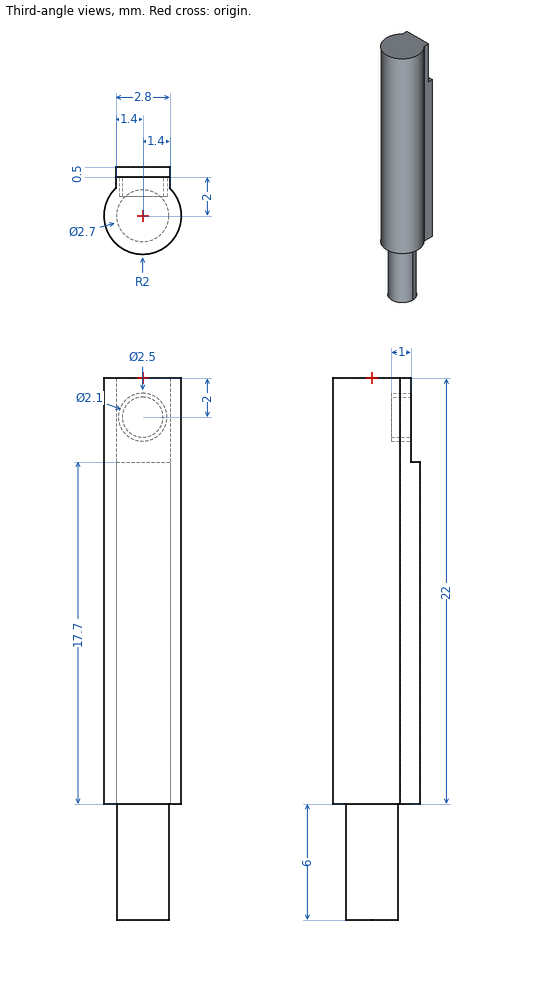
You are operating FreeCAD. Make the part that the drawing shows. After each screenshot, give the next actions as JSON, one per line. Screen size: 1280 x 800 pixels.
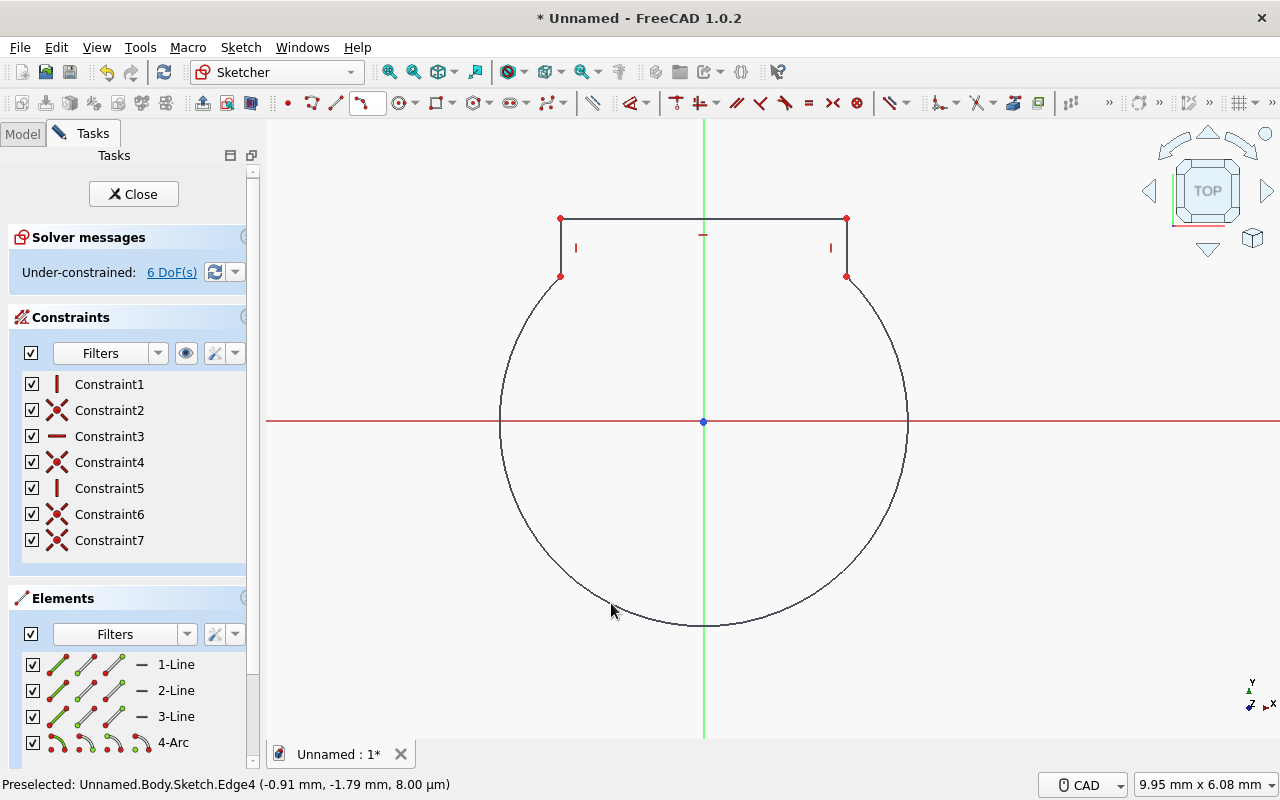
{"action": "left_click_drag", "start_coordinate": [694, 411], "coordinate": [714, 432]}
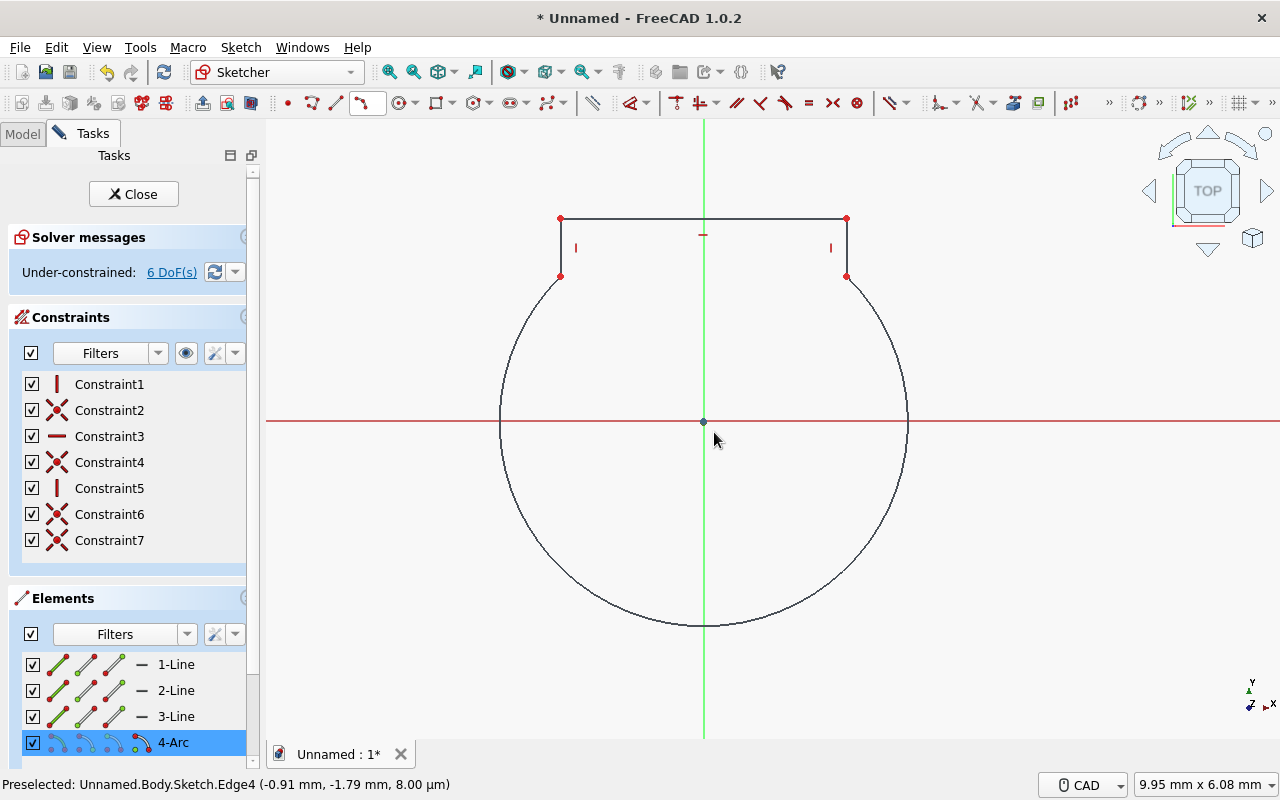
{"action": "left_click", "coordinate": [676, 104]}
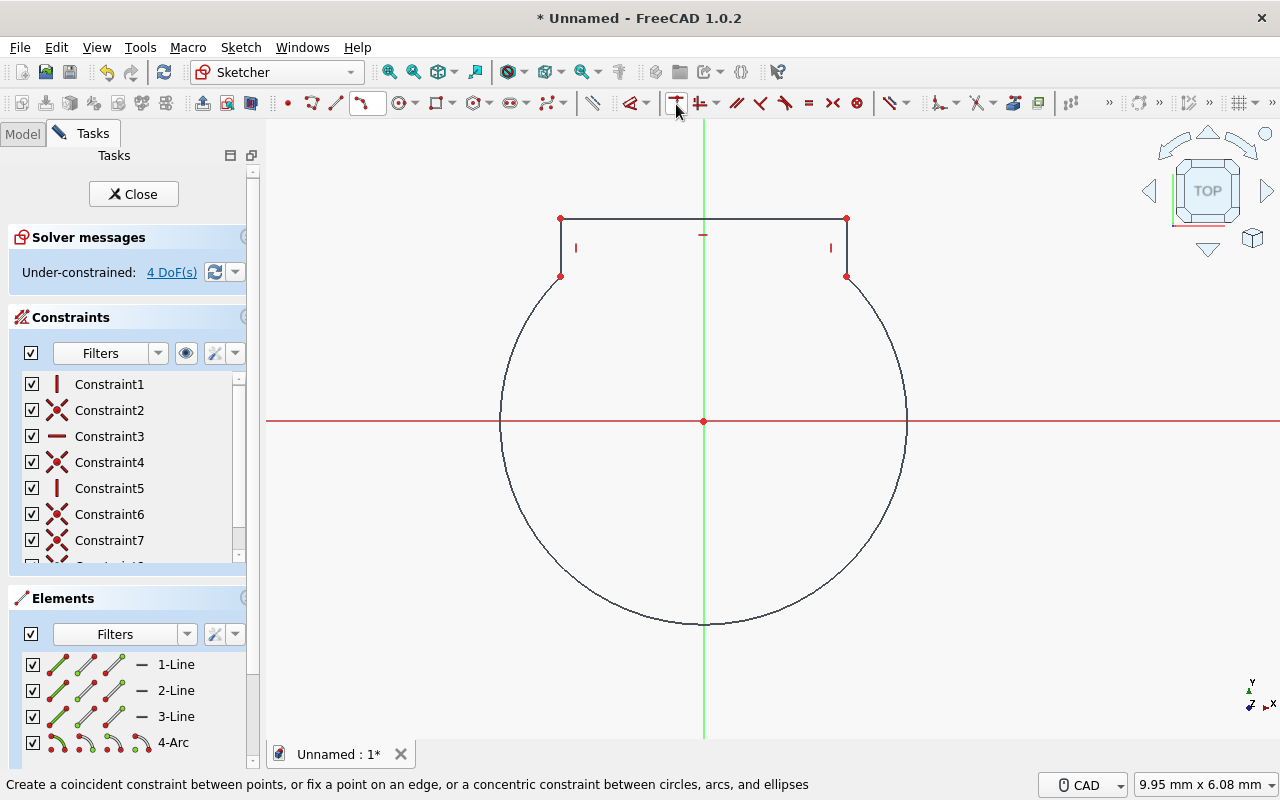
{"action": "left_click", "coordinate": [539, 540]}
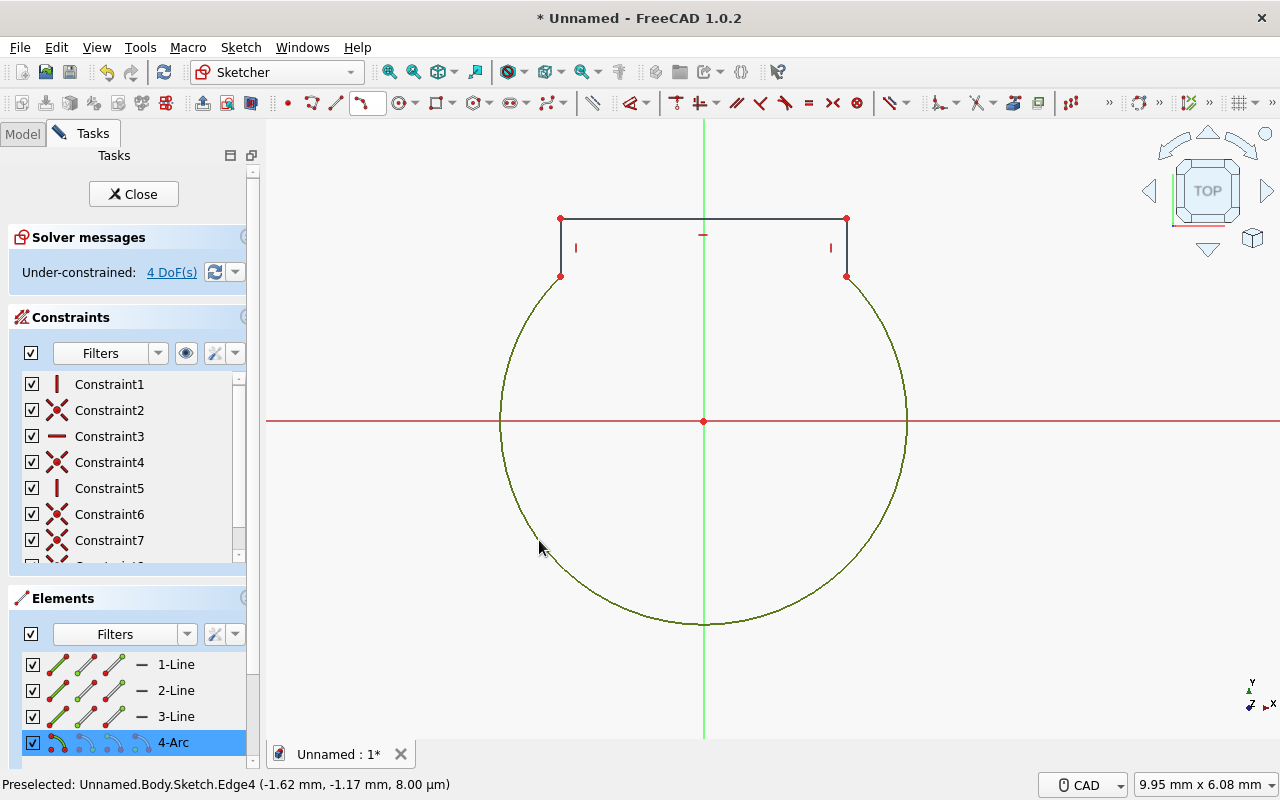
{"action": "left_click", "coordinate": [648, 104]}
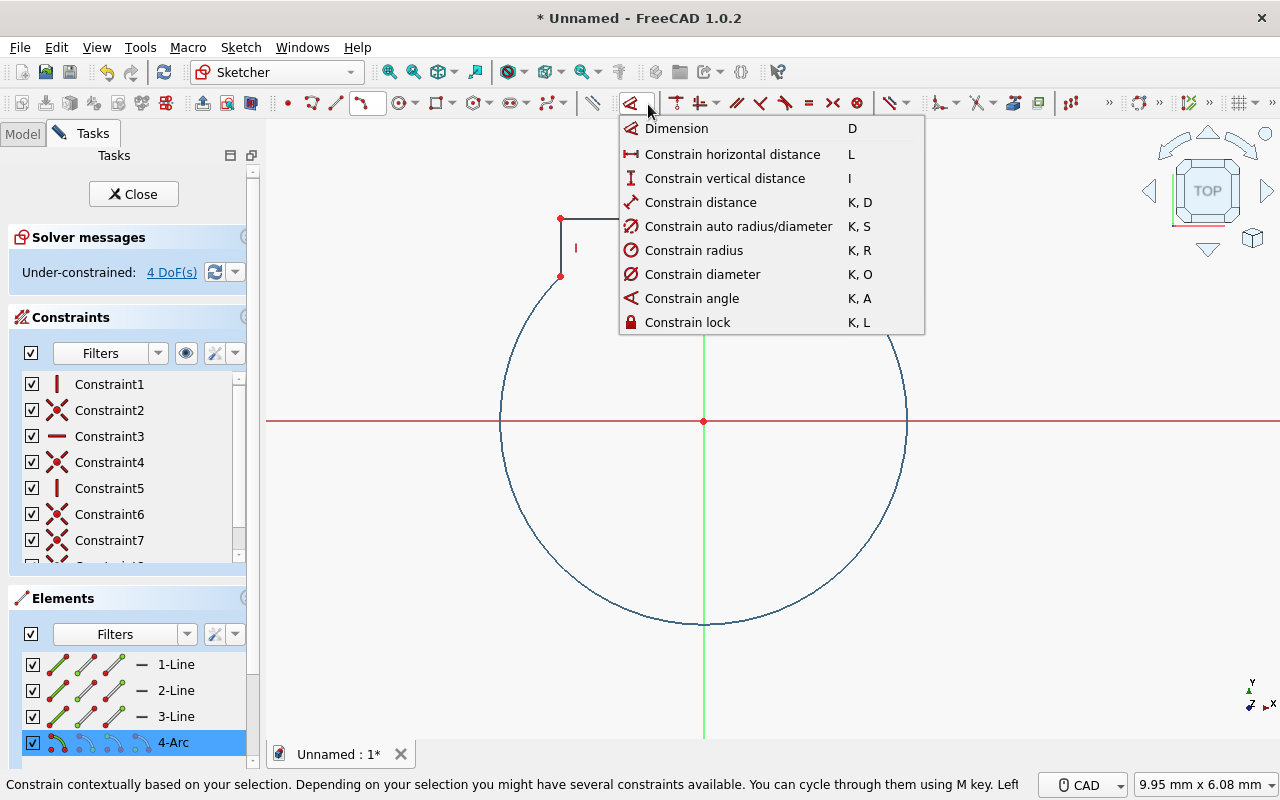
{"action": "left_click", "coordinate": [772, 250]}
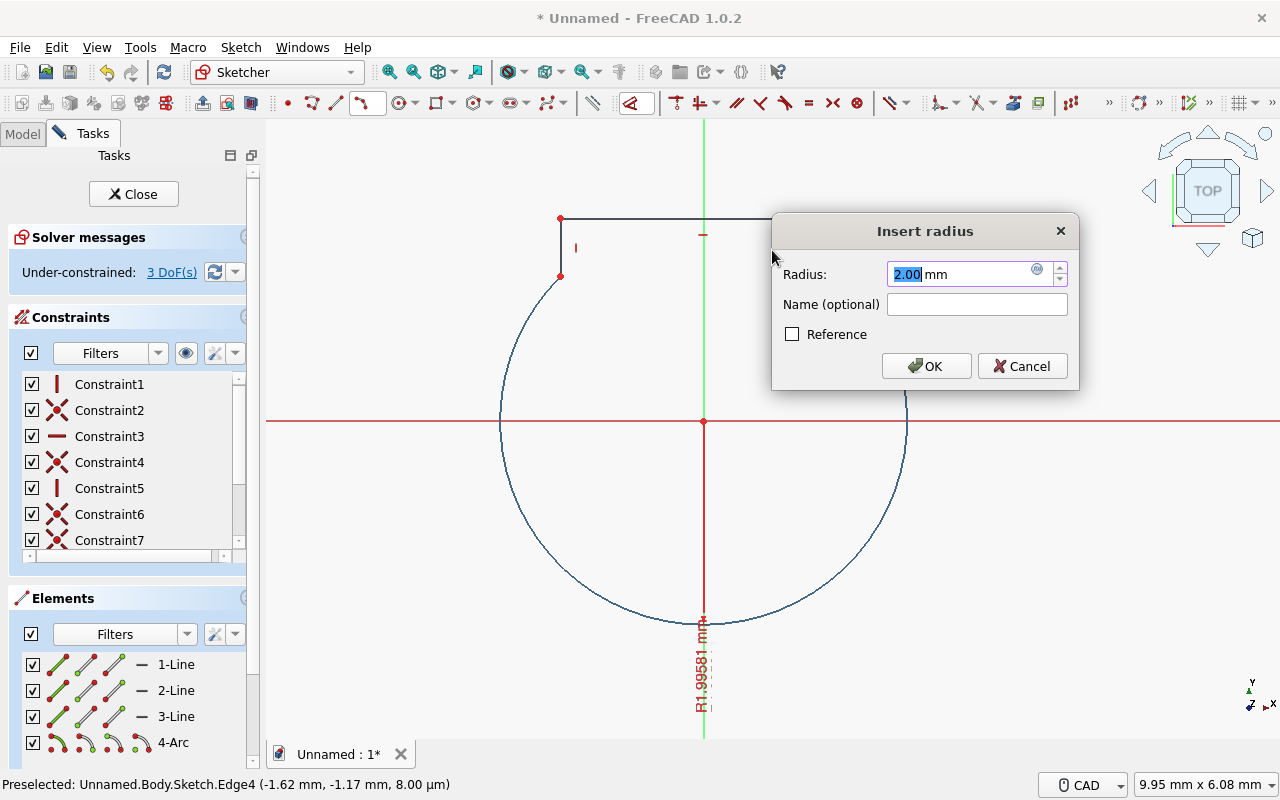
{"action": "type", "text": "2"}
{"action": "key", "text": "Return"}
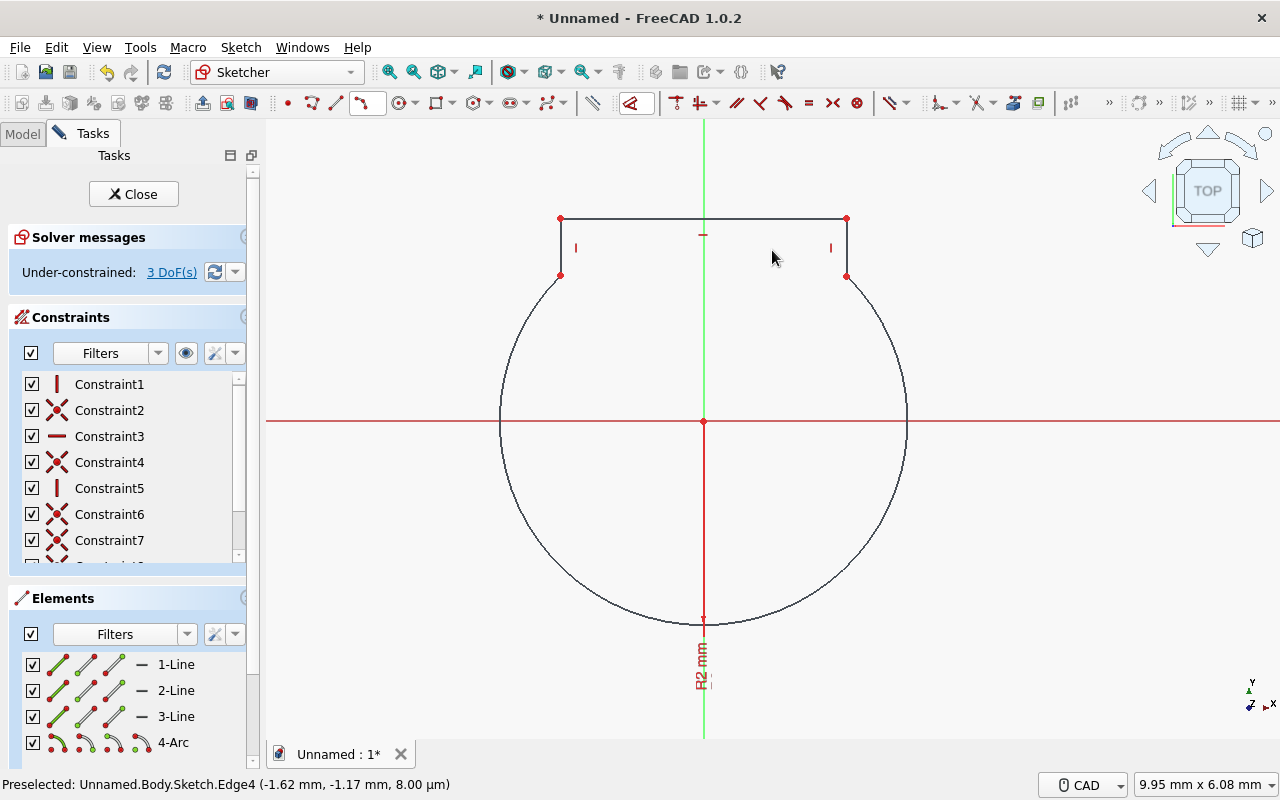
{"action": "left_click", "coordinate": [847, 219]}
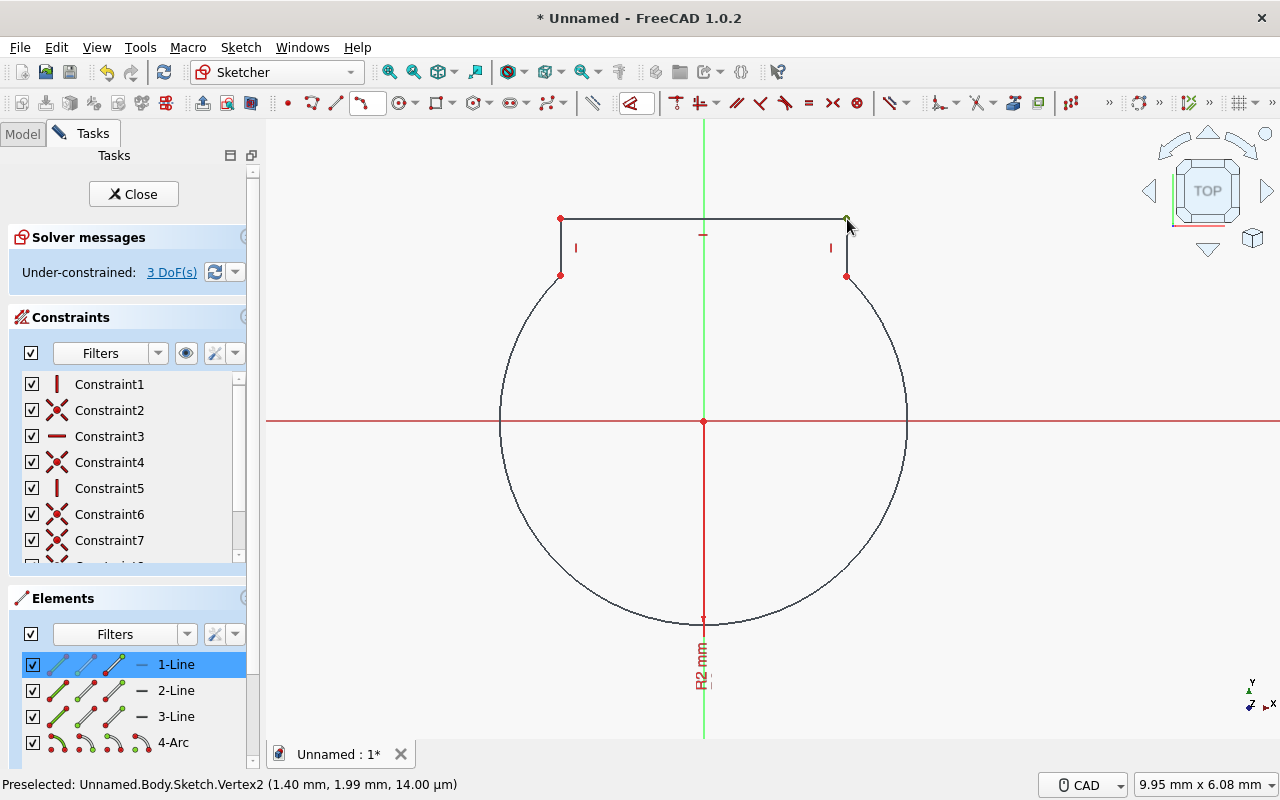
{"action": "left_click", "coordinate": [648, 104]}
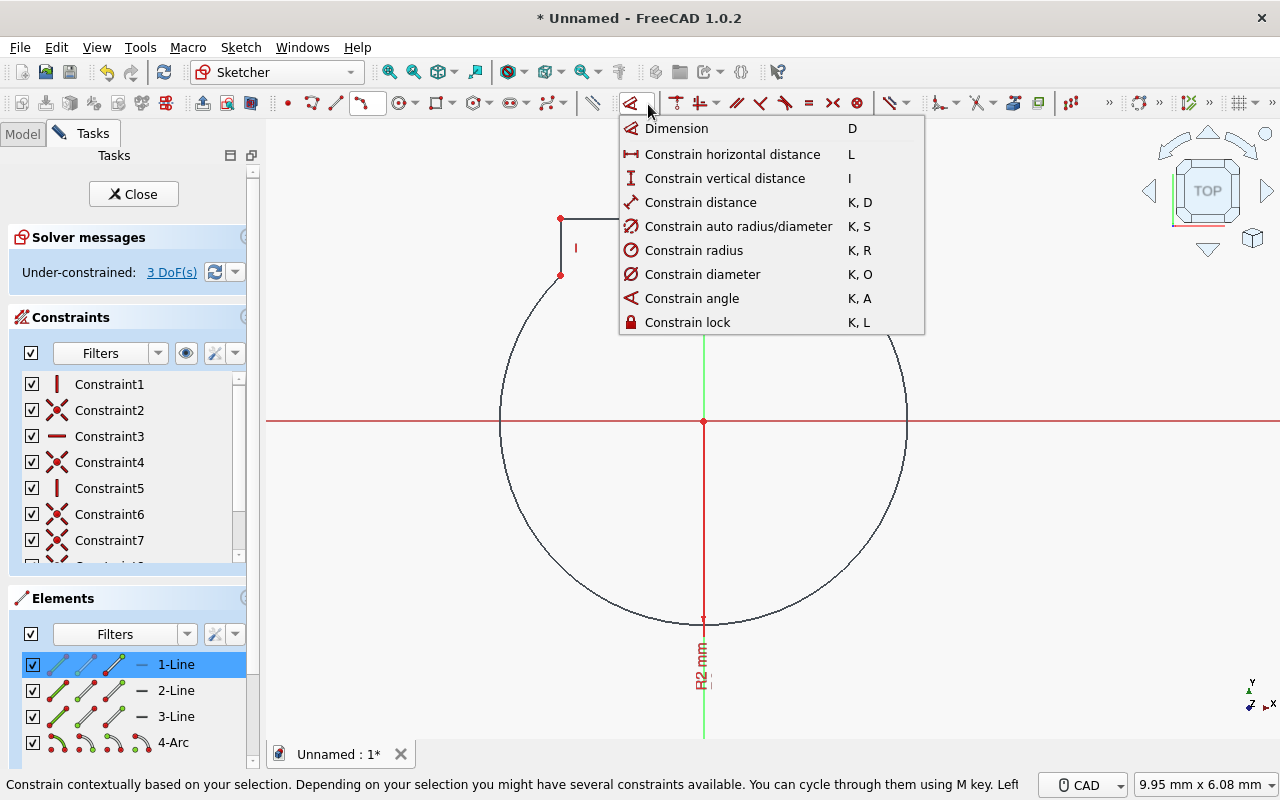
{"action": "left_click", "coordinate": [772, 178]}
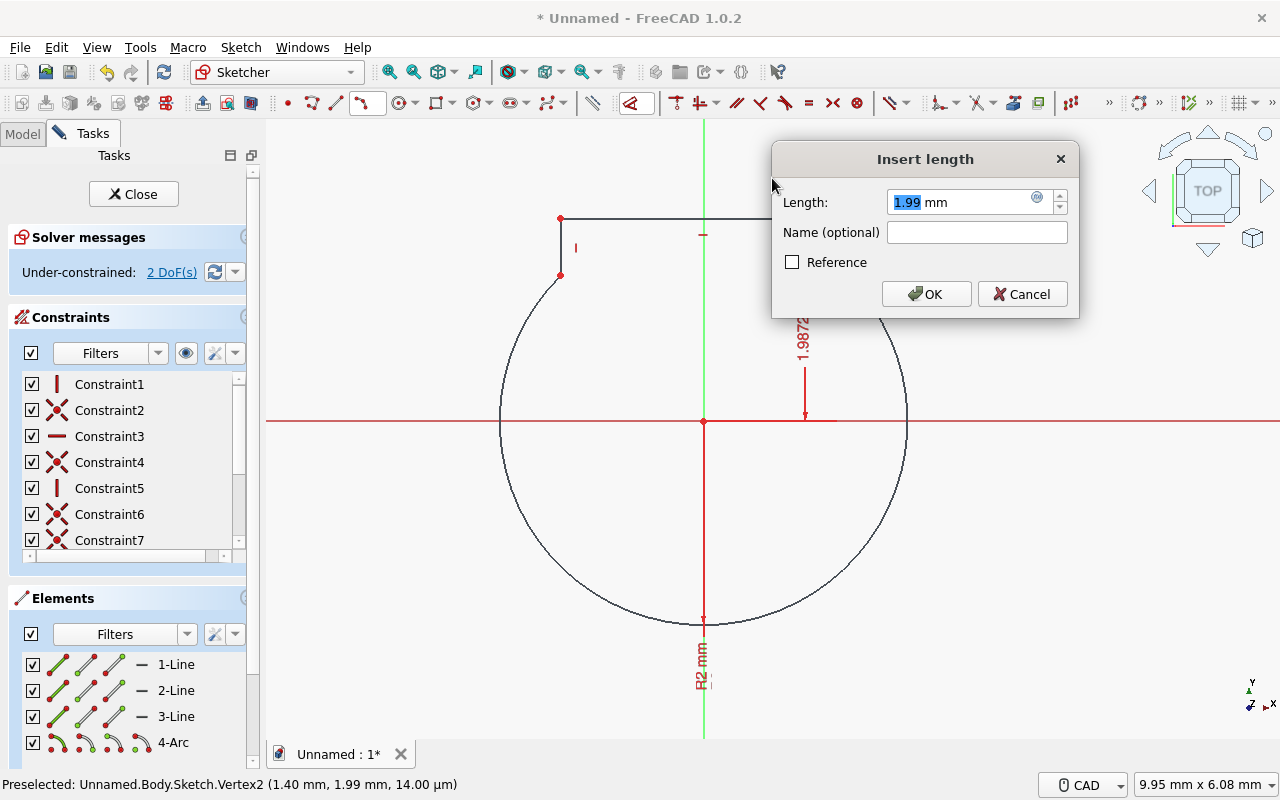
{"action": "type", "text": "2"}
{"action": "key", "text": "Return"}